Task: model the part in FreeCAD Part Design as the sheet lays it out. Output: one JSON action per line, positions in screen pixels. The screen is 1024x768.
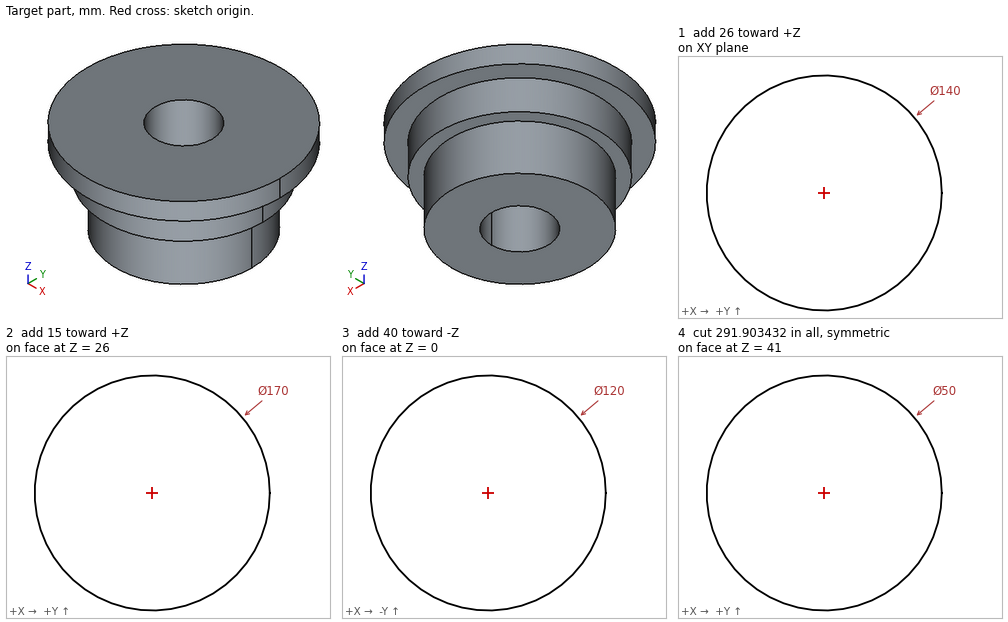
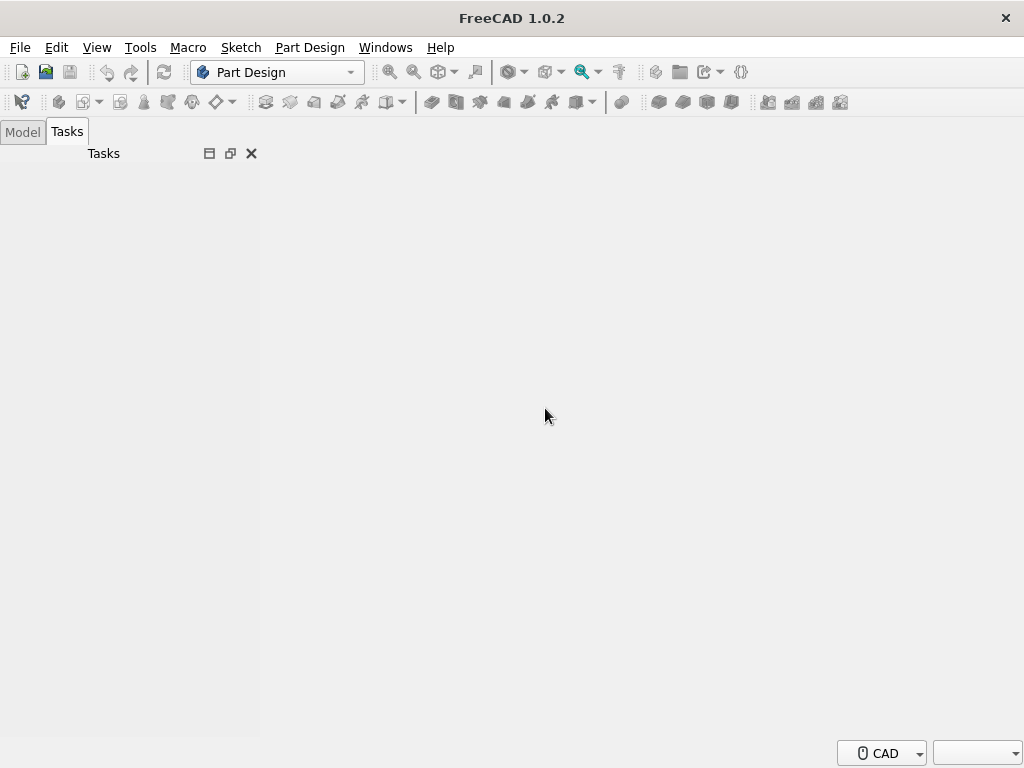
{"action": "key", "text": "ctrl+n"}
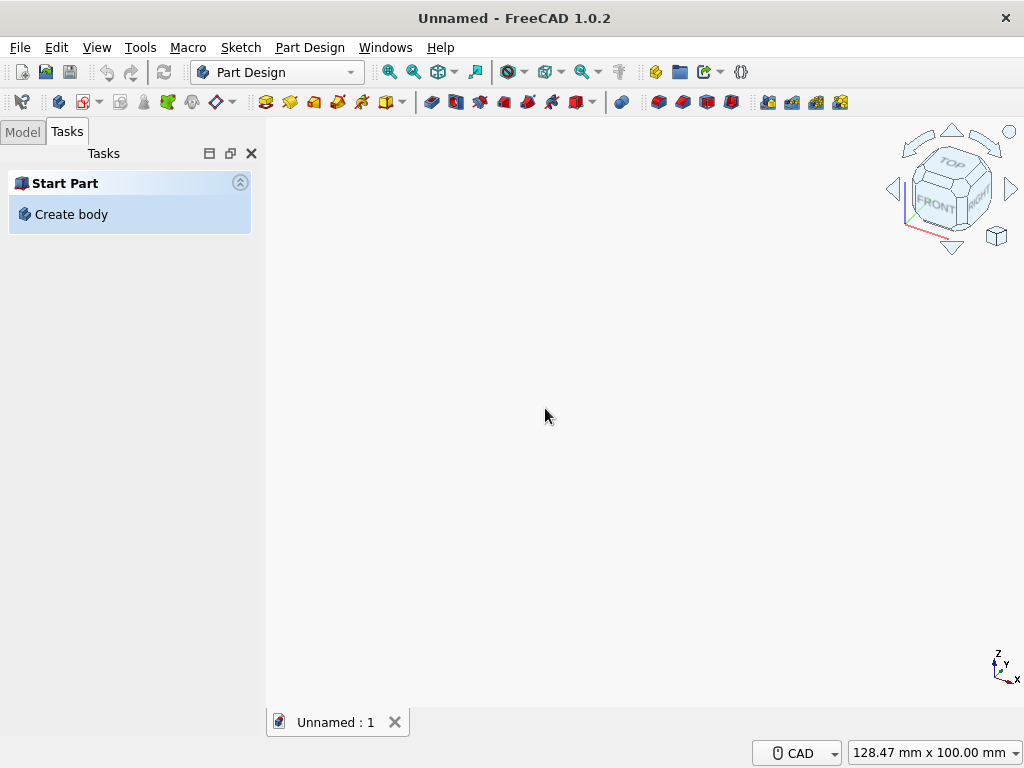
{"action": "left_click", "coordinate": [84, 102]}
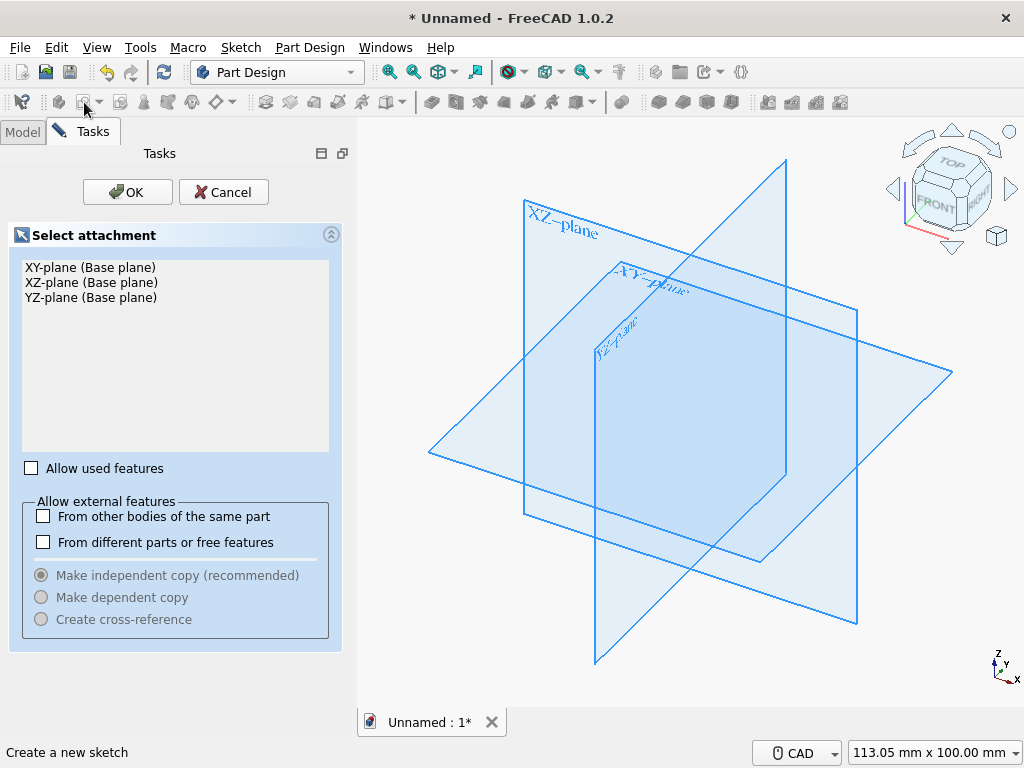
{"action": "left_click", "coordinate": [82, 268]}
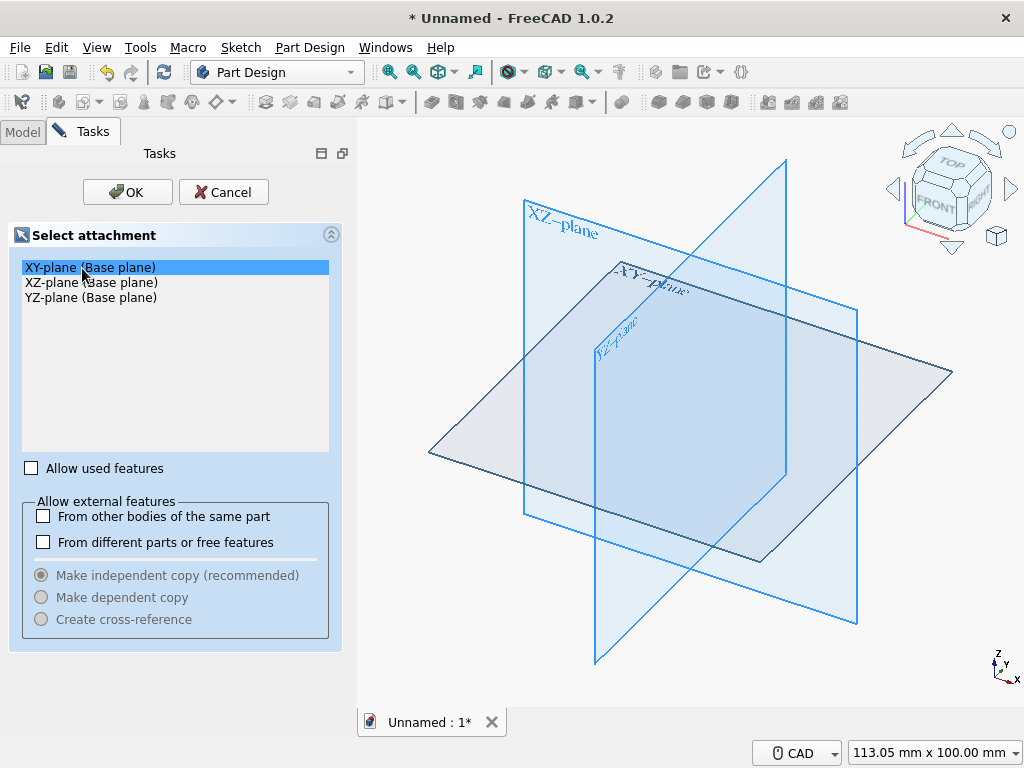
{"action": "left_click", "coordinate": [128, 192]}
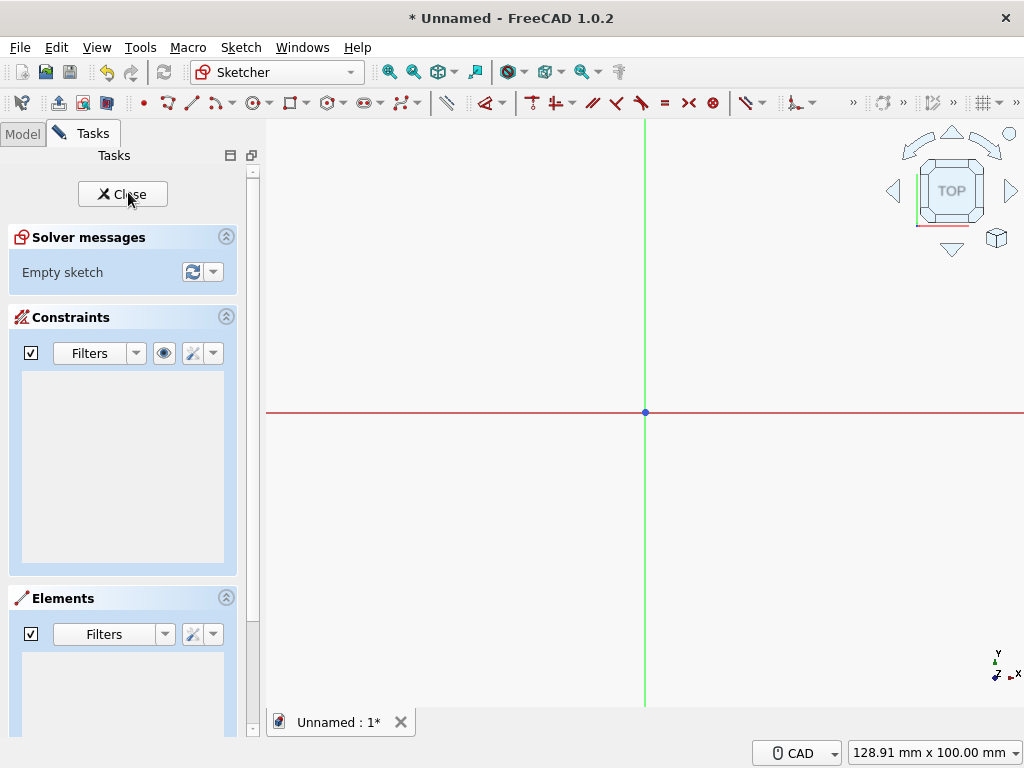
{"action": "scroll", "coordinate": [521, 413], "scroll_direction": "down", "scroll_amount": 4}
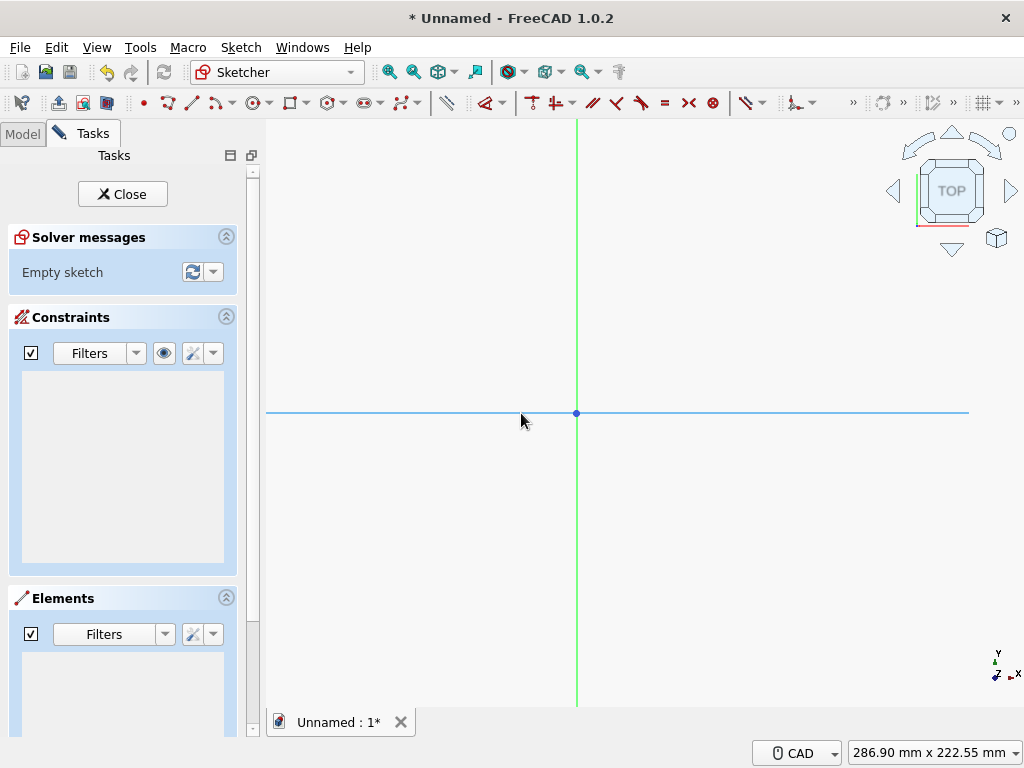
{"action": "key", "text": "g c"}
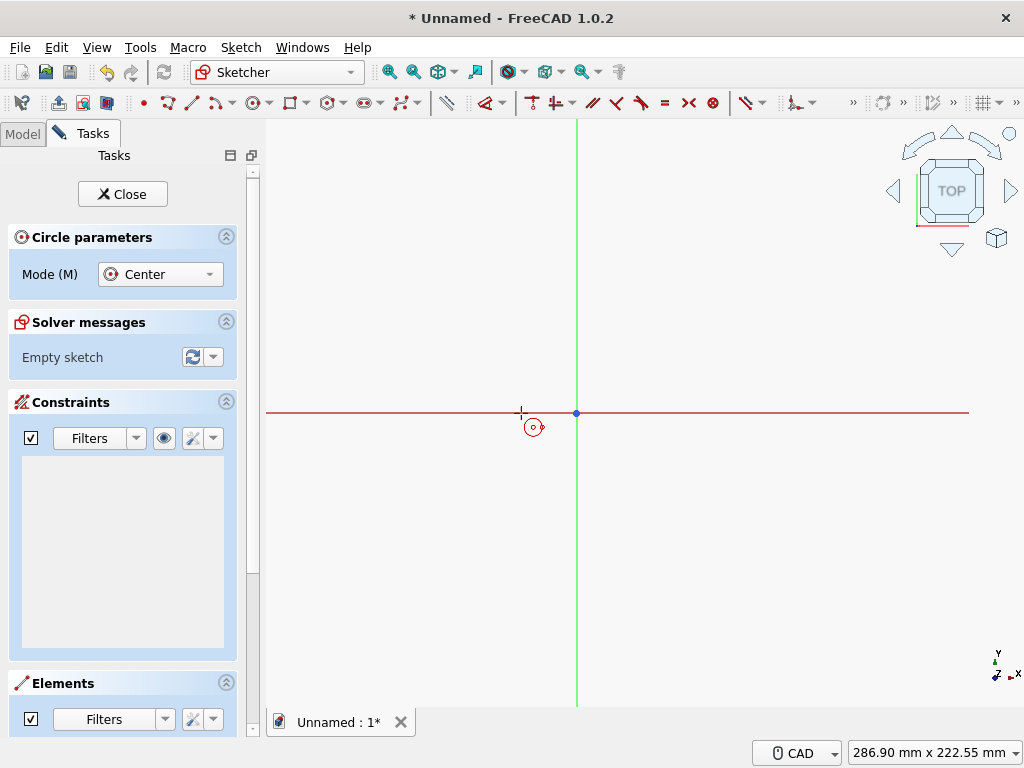
{"action": "left_click", "coordinate": [577, 413]}
{"action": "left_click", "coordinate": [708, 283]}
{"action": "key", "text": "Escape"}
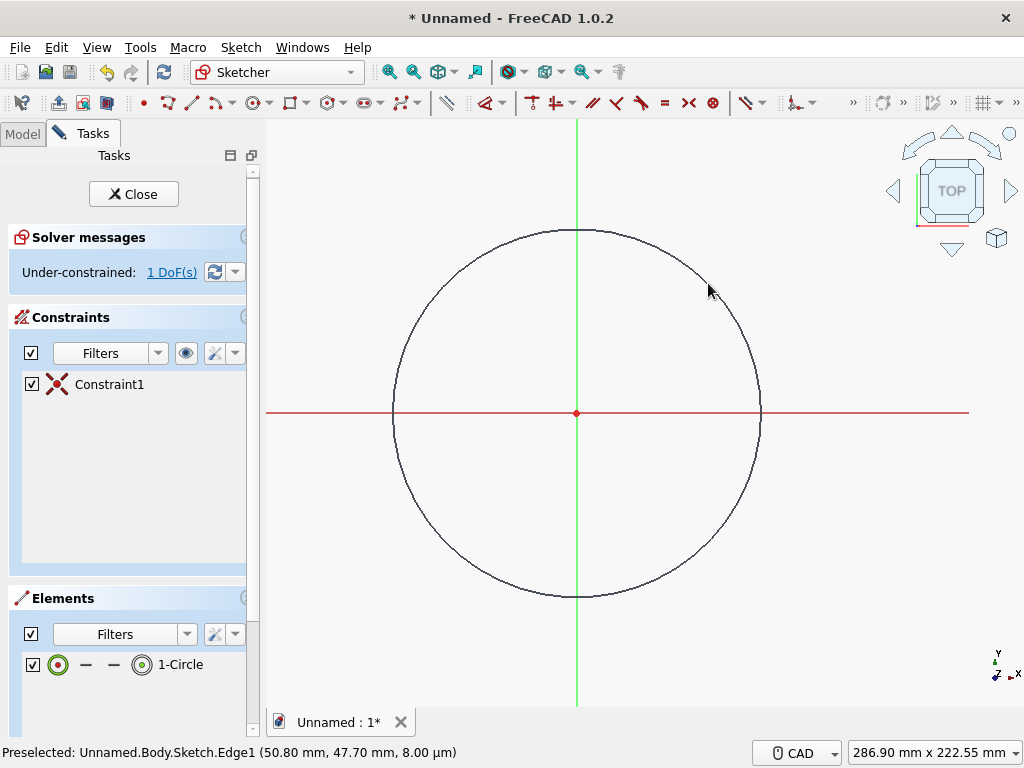
{"action": "key", "text": "d"}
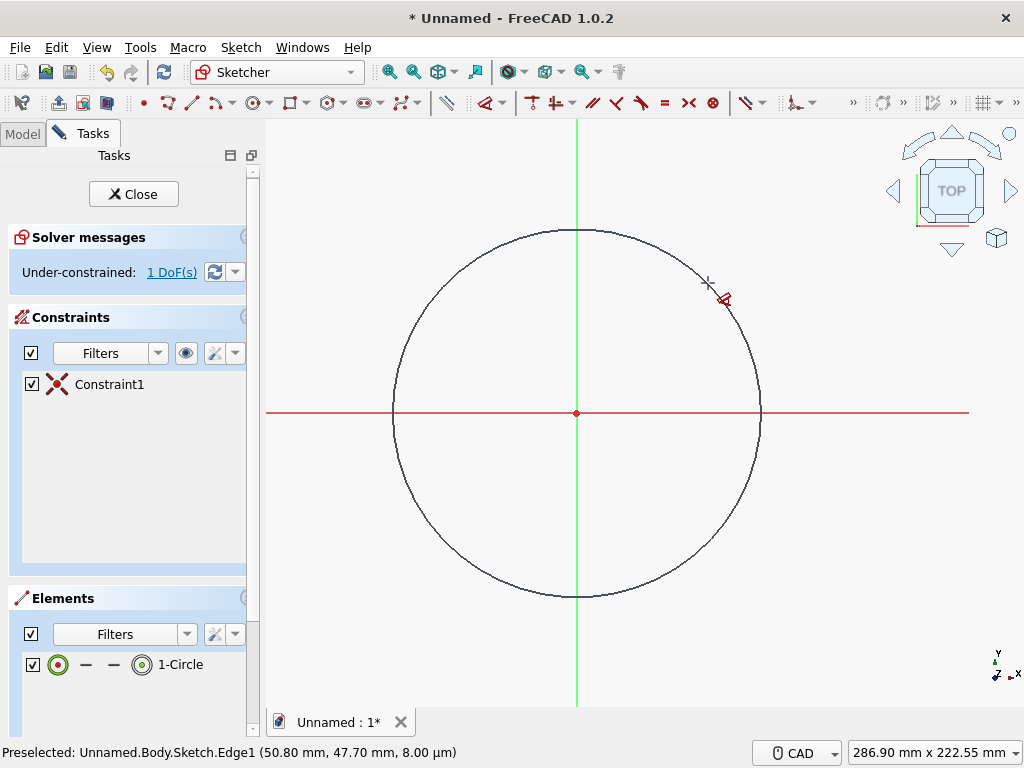
{"action": "left_click", "coordinate": [707, 283]}
{"action": "left_click", "coordinate": [730, 260]}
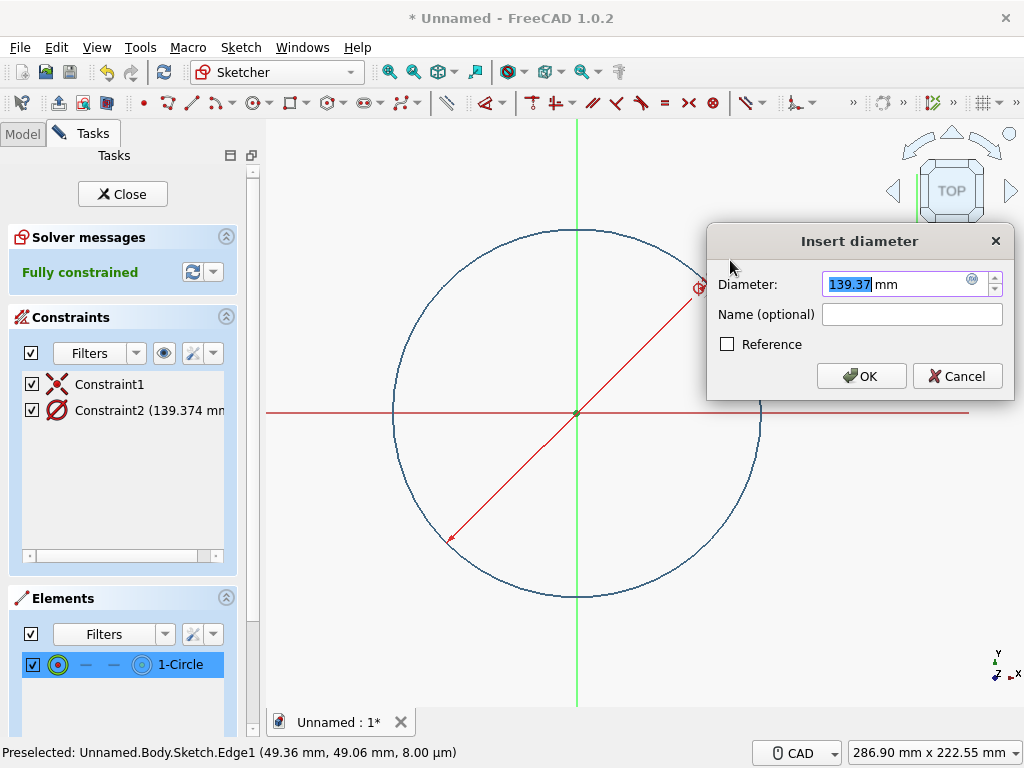
{"action": "type", "text": "140"}
{"action": "key", "text": "Return"}
{"action": "key", "text": "Escape"}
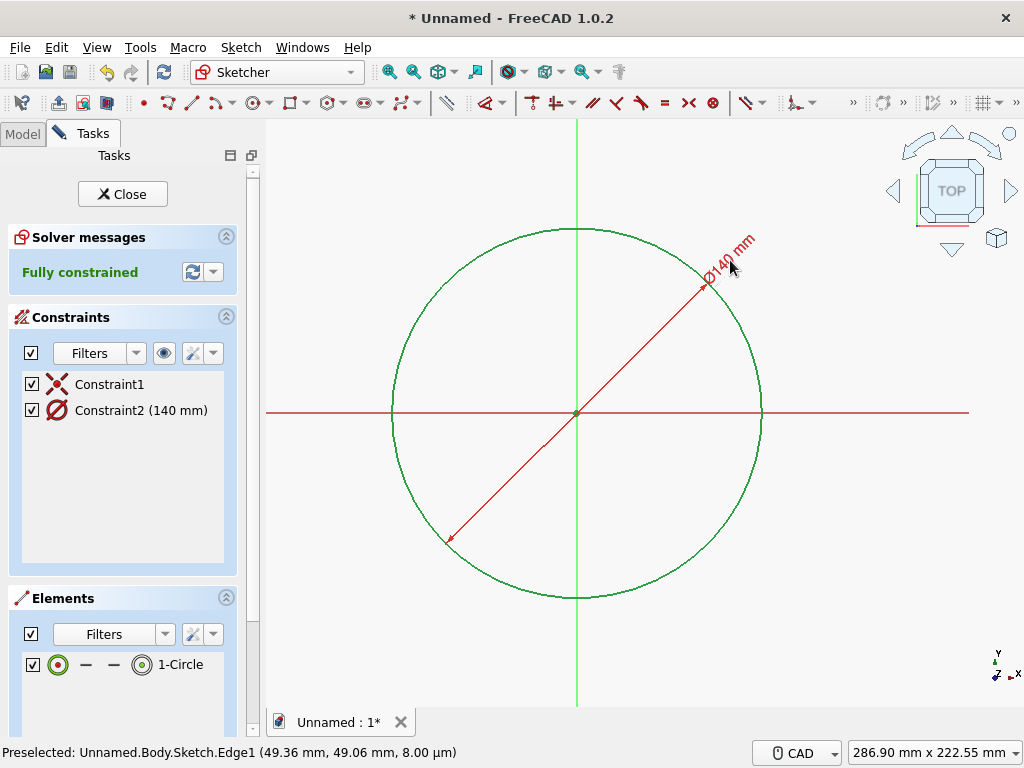
{"action": "left_click", "coordinate": [123, 194]}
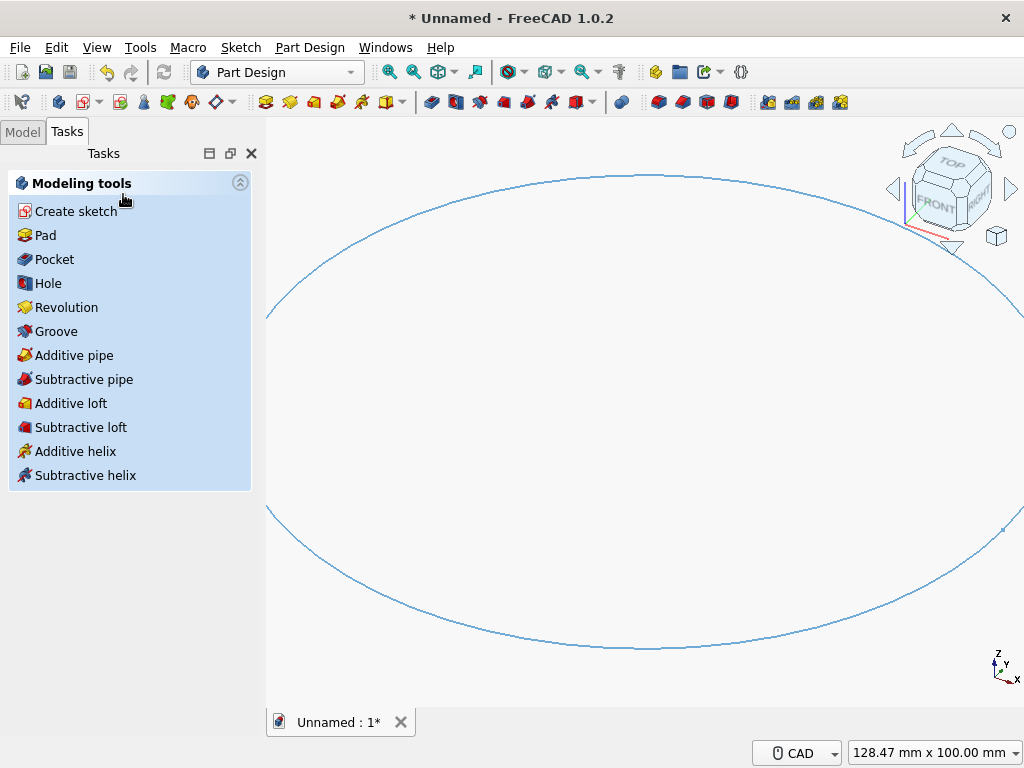
{"action": "left_click", "coordinate": [266, 102]}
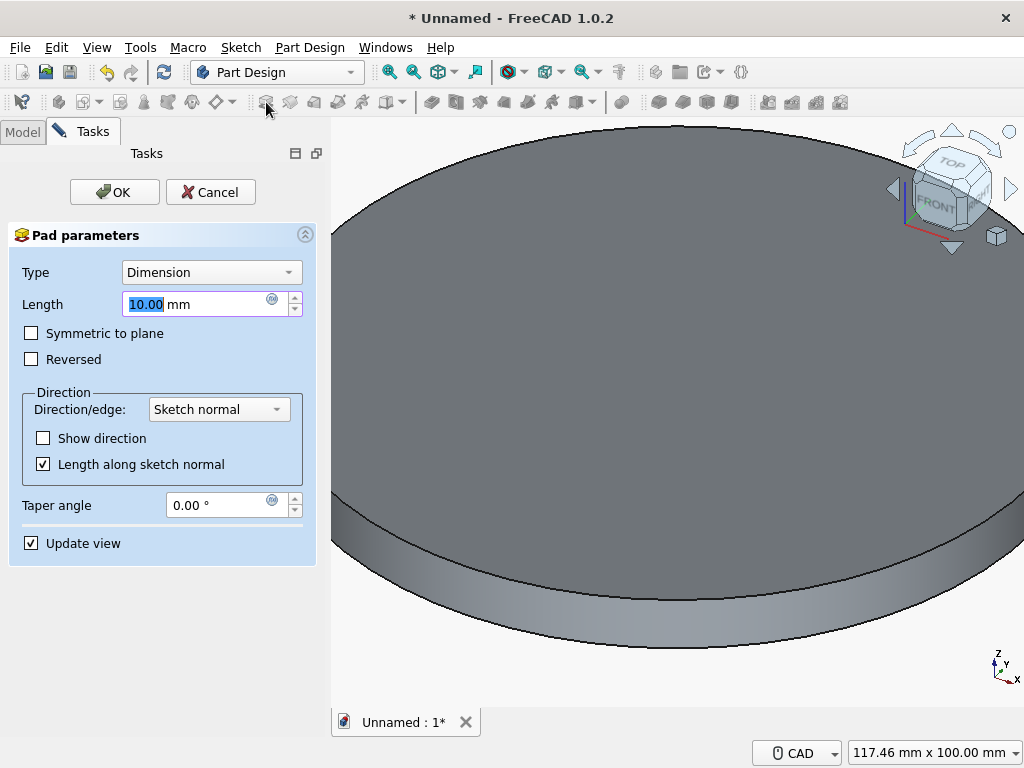
{"action": "type", "text": "26"}
{"action": "key", "text": "Tab"}